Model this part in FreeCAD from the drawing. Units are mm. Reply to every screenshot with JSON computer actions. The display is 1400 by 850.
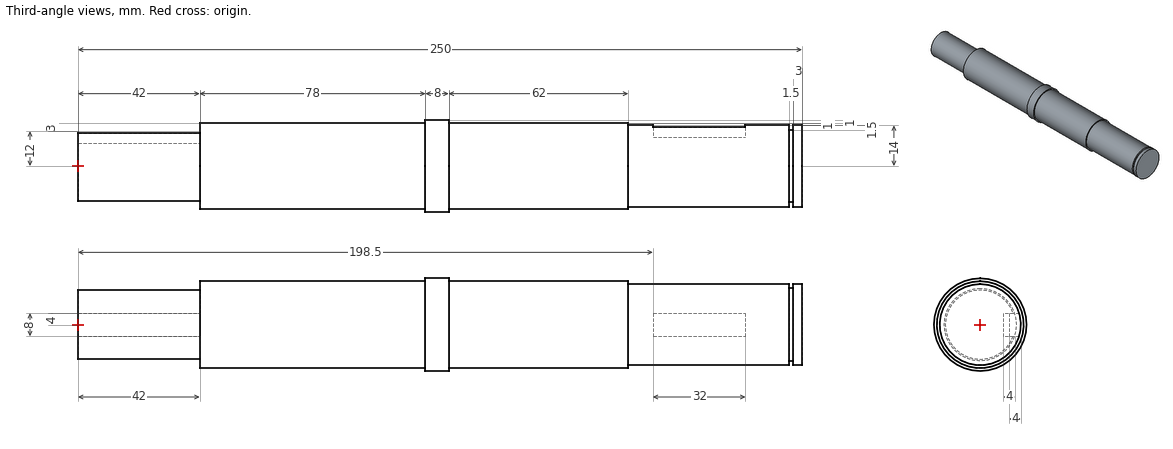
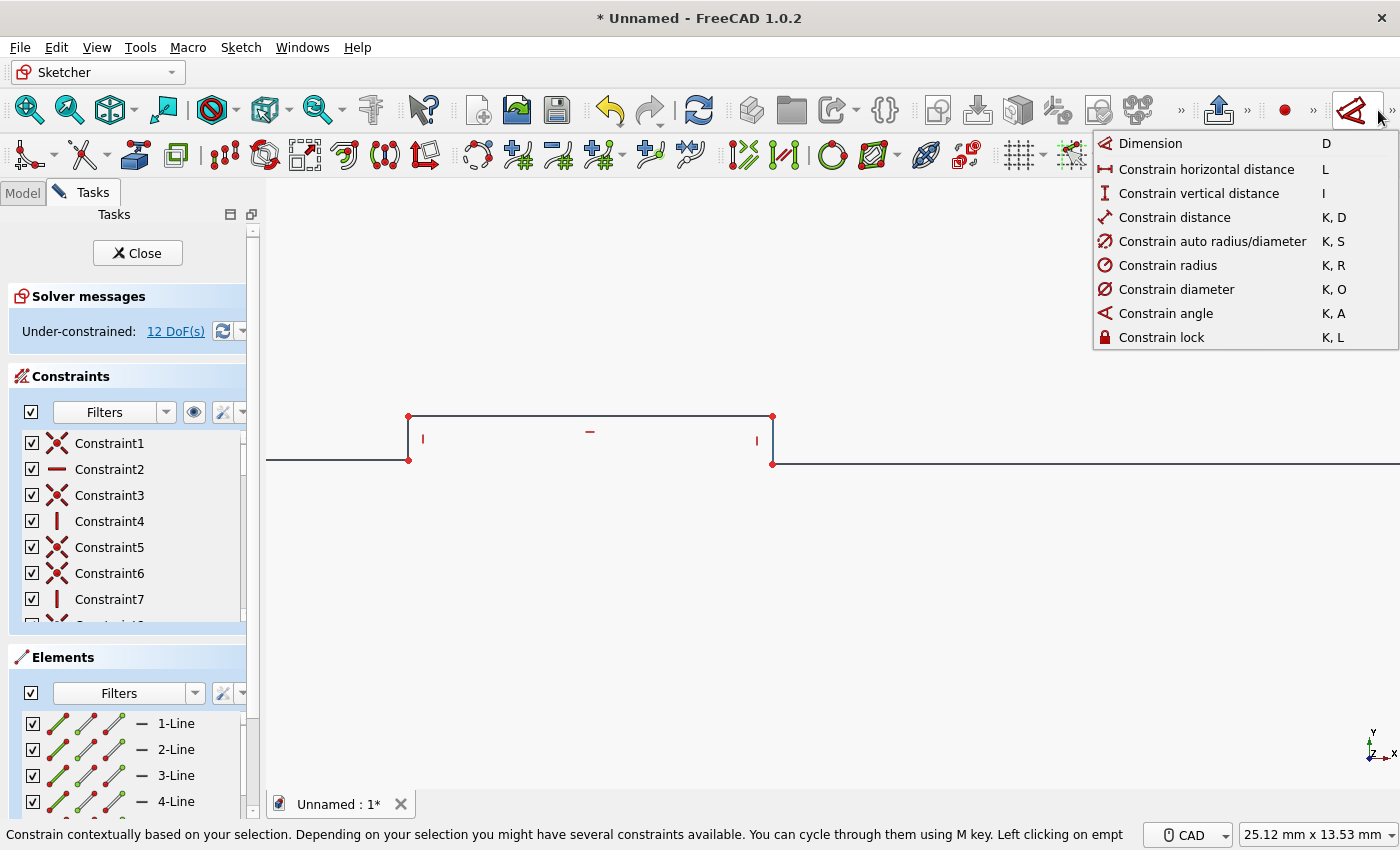
{"action": "left_click", "coordinate": [1246, 193]}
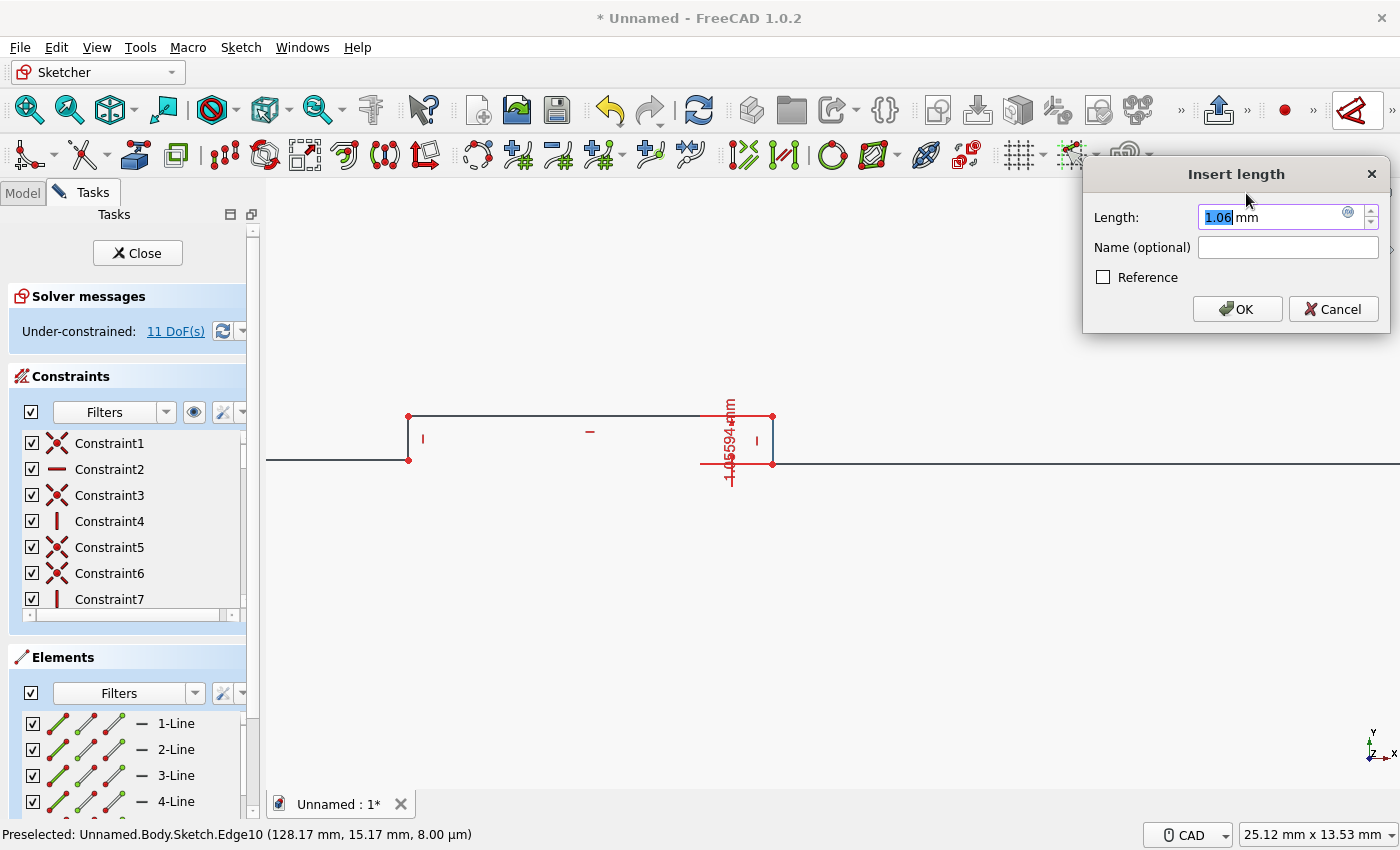
{"action": "type", "text": "1"}
{"action": "key", "text": "Return"}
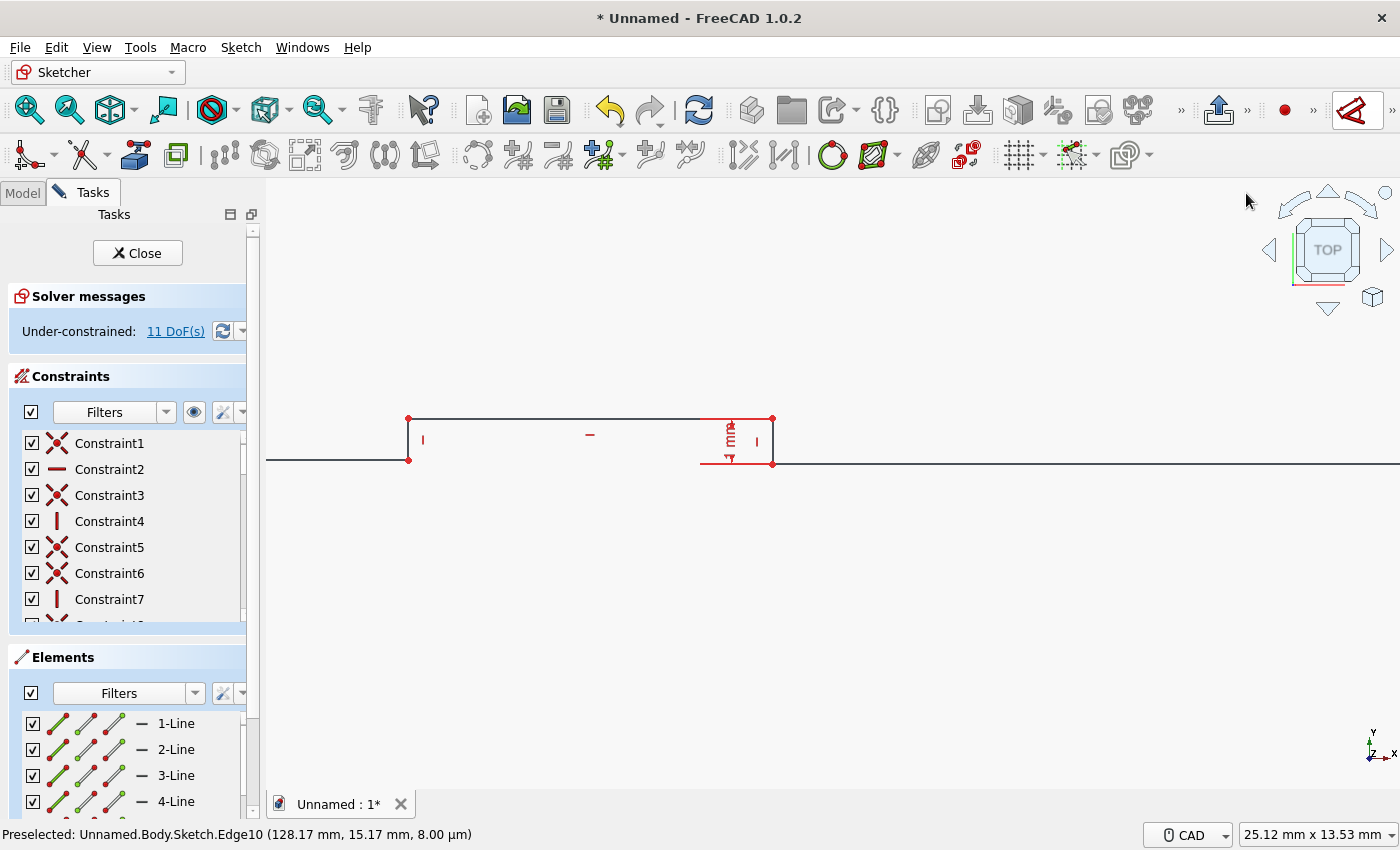
{"action": "scroll", "coordinate": [773, 465], "scroll_direction": "down", "scroll_amount": 14}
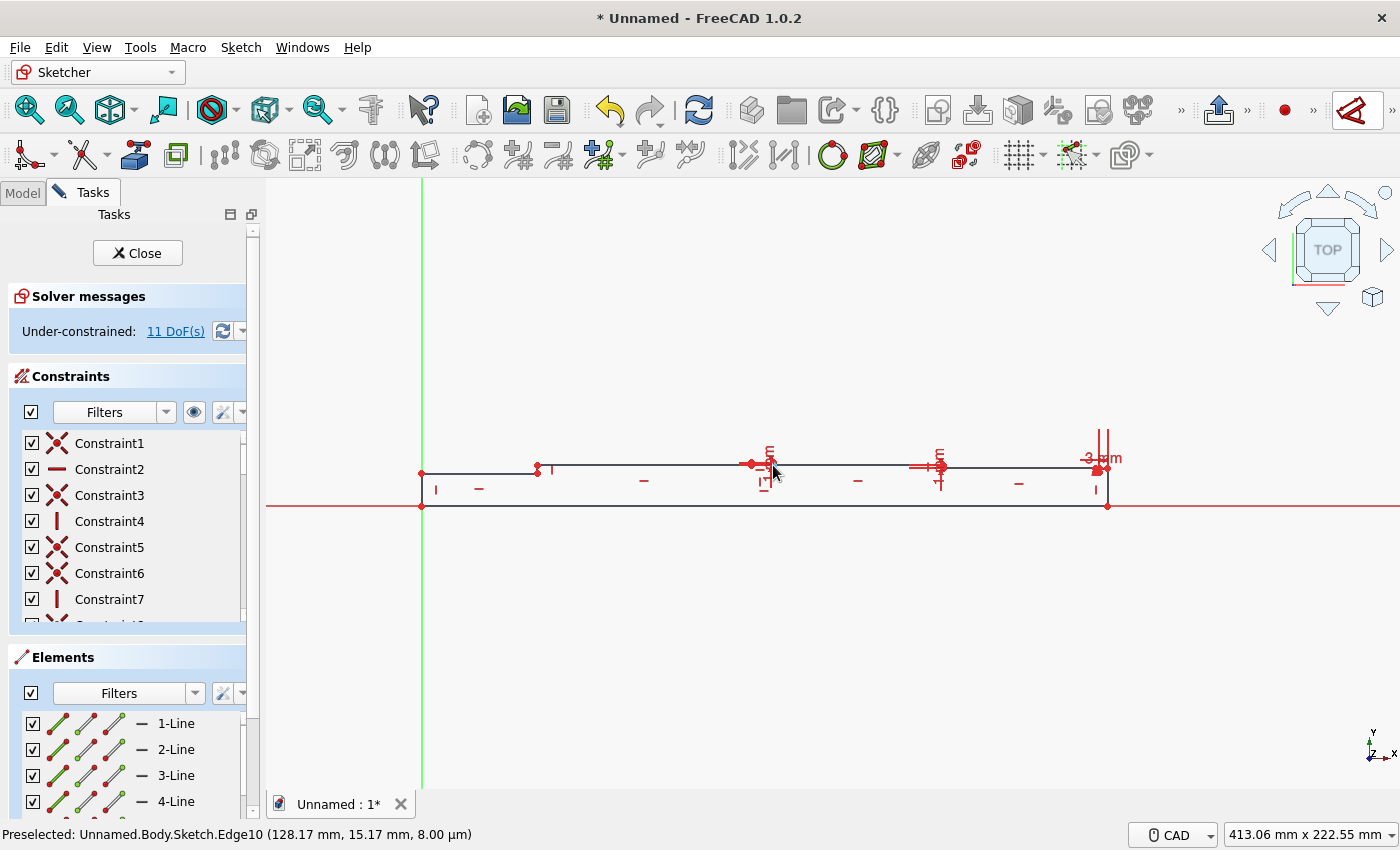
{"action": "scroll", "coordinate": [767, 463], "scroll_direction": "up", "scroll_amount": 4}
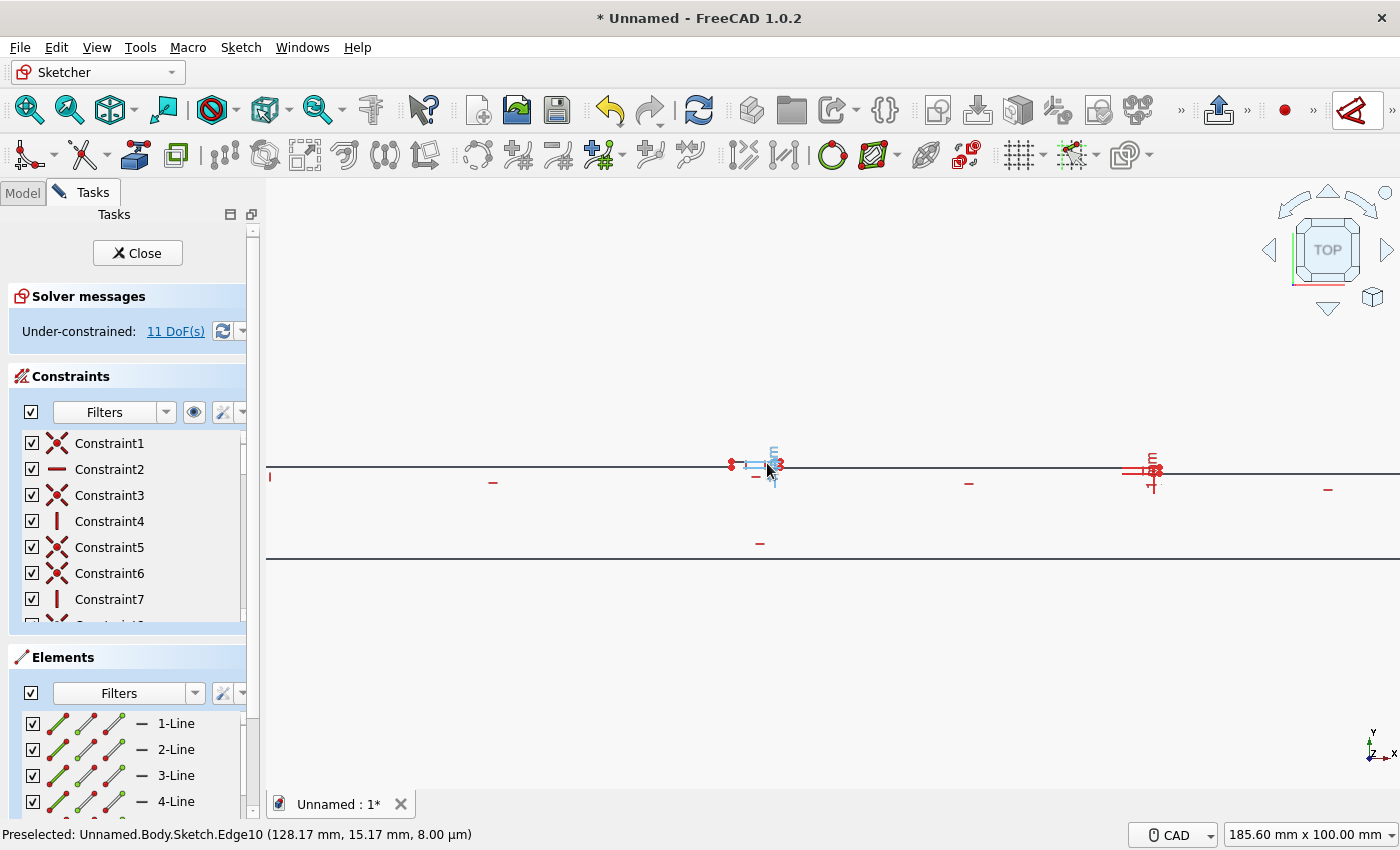
{"action": "left_click", "coordinate": [756, 462]}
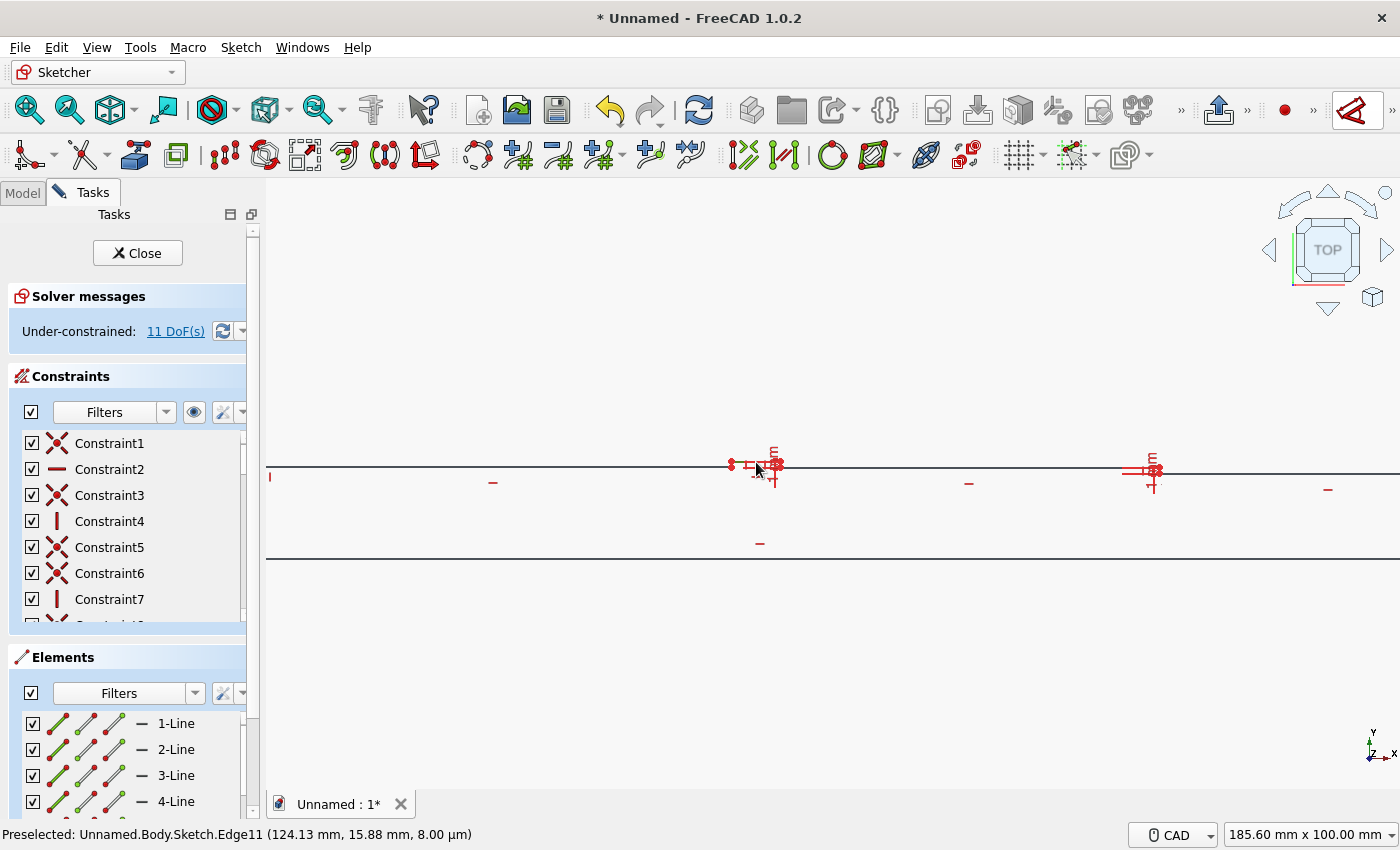
{"action": "key", "text": "l"}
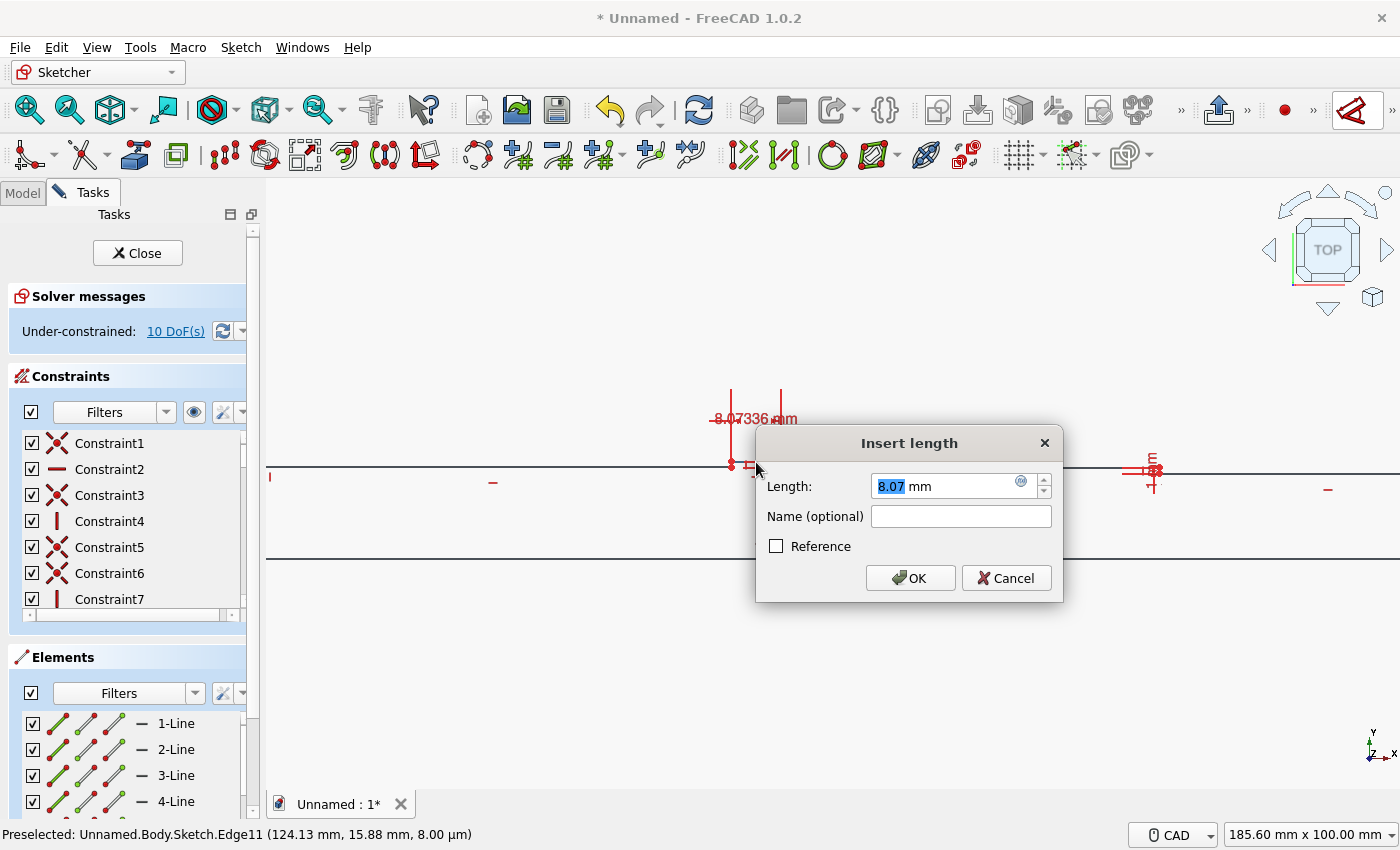
{"action": "type", "text": "8"}
{"action": "key", "text": "Return"}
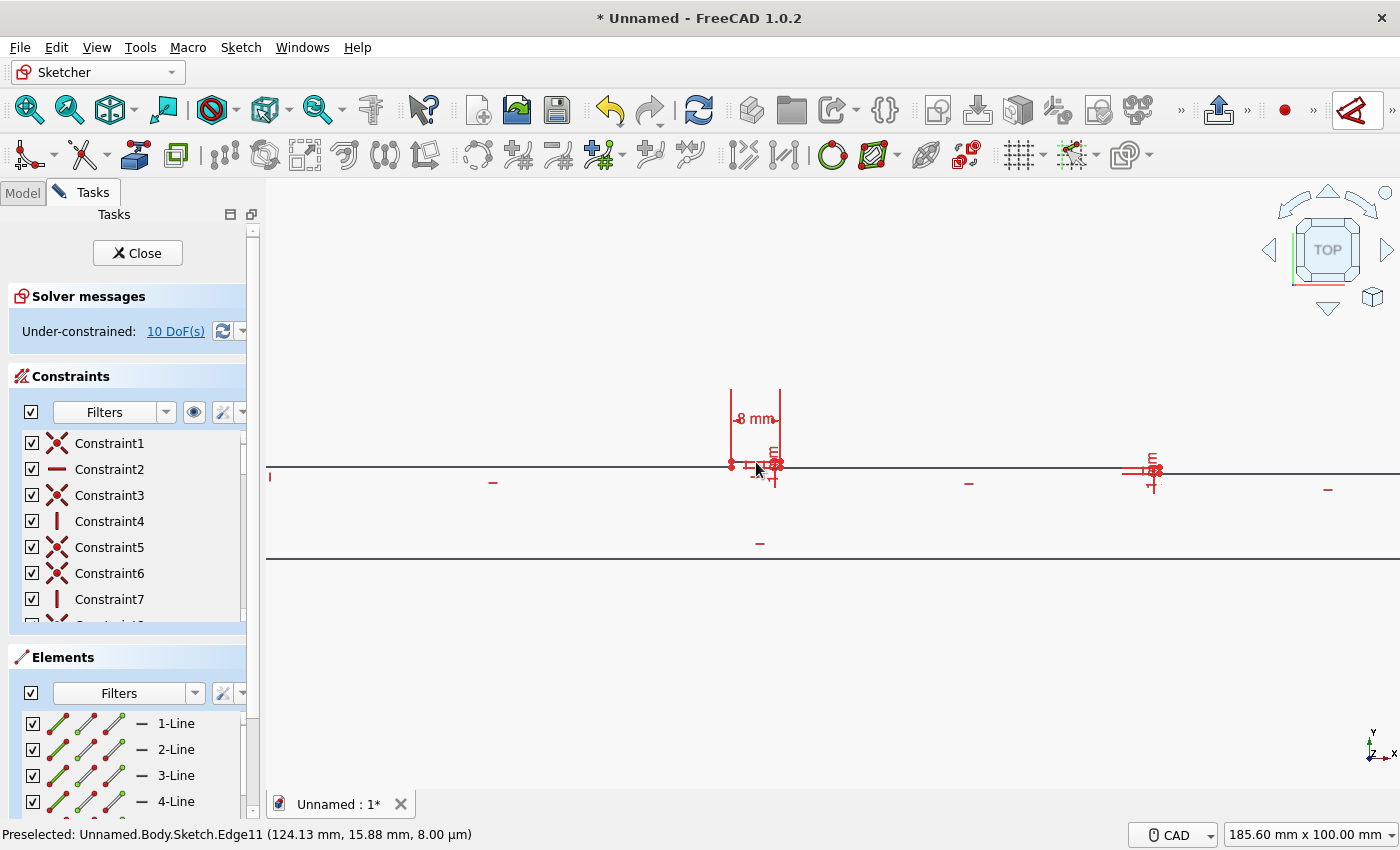
{"action": "scroll", "coordinate": [731, 464], "scroll_direction": "up", "scroll_amount": 10}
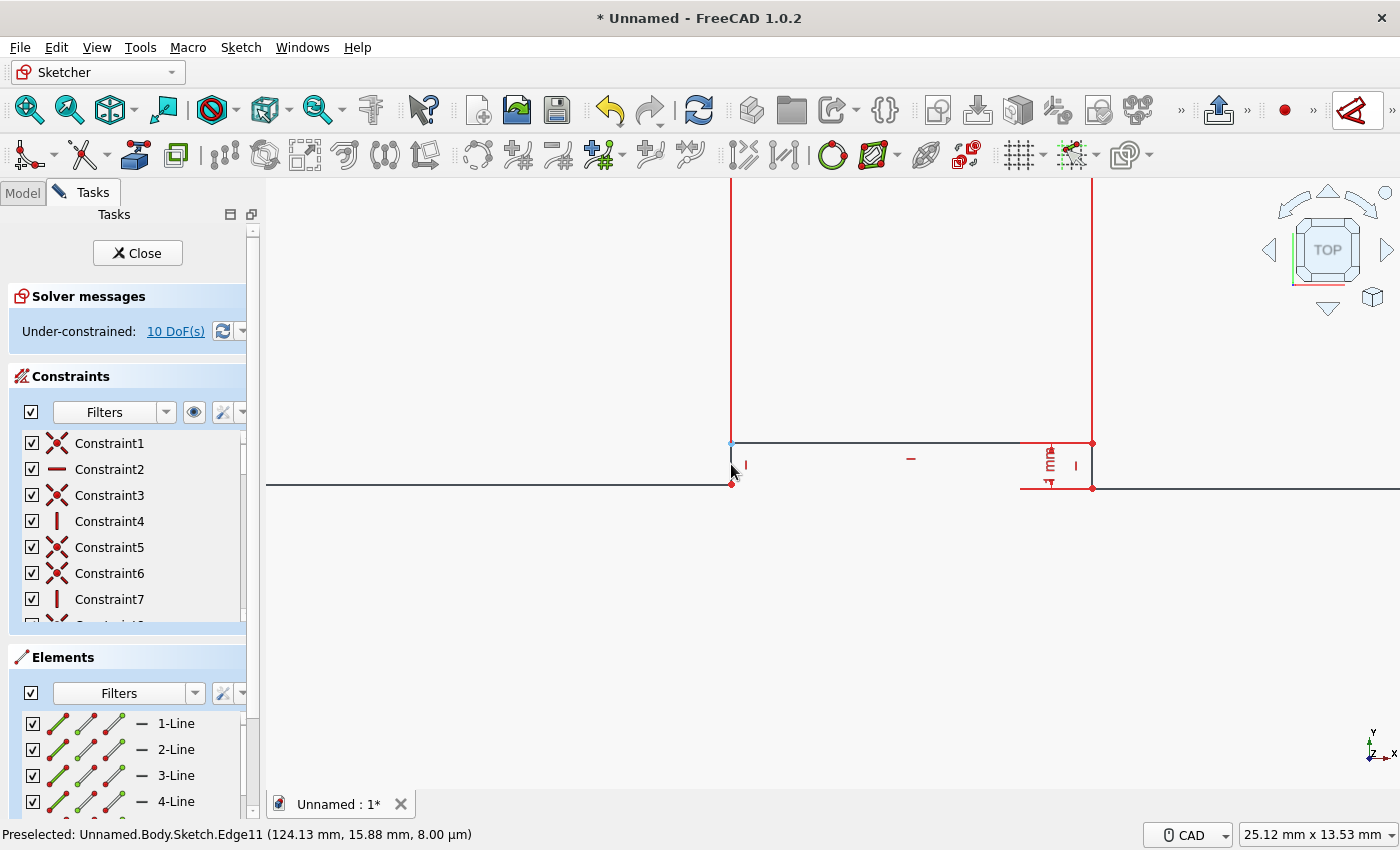
{"action": "left_click", "coordinate": [731, 464]}